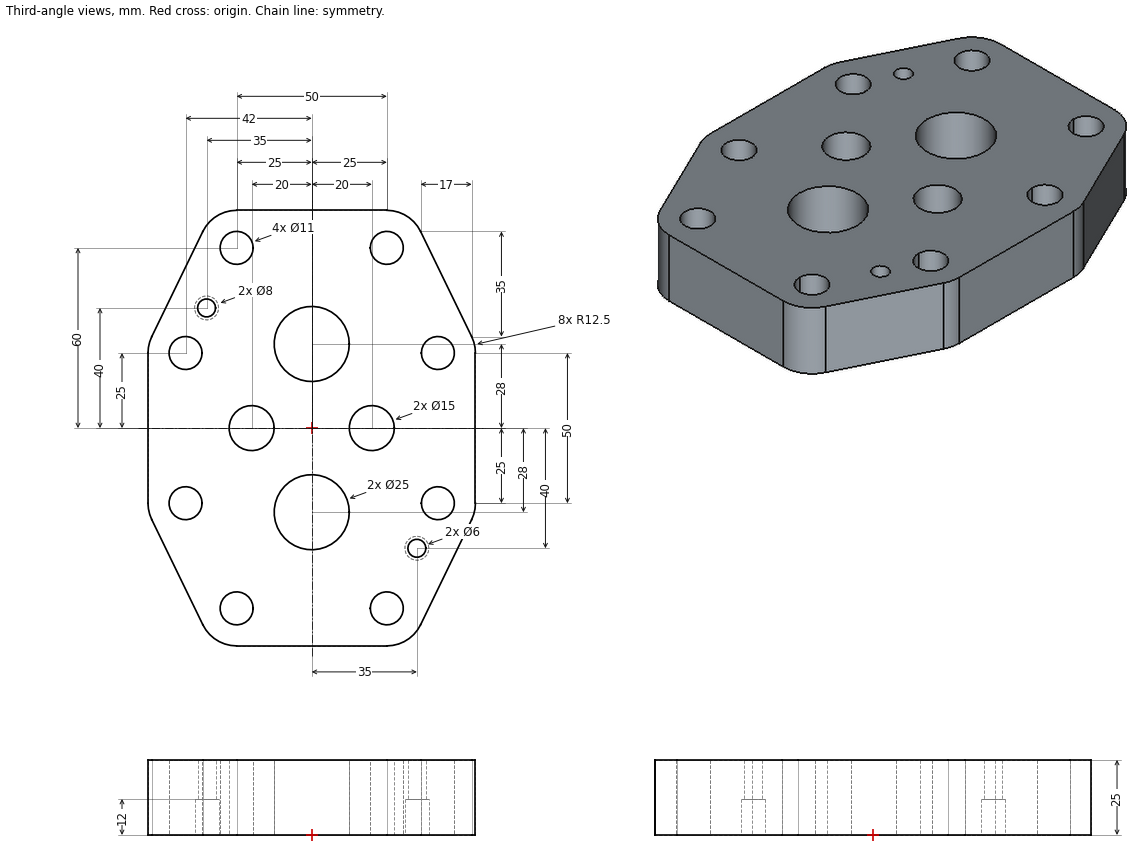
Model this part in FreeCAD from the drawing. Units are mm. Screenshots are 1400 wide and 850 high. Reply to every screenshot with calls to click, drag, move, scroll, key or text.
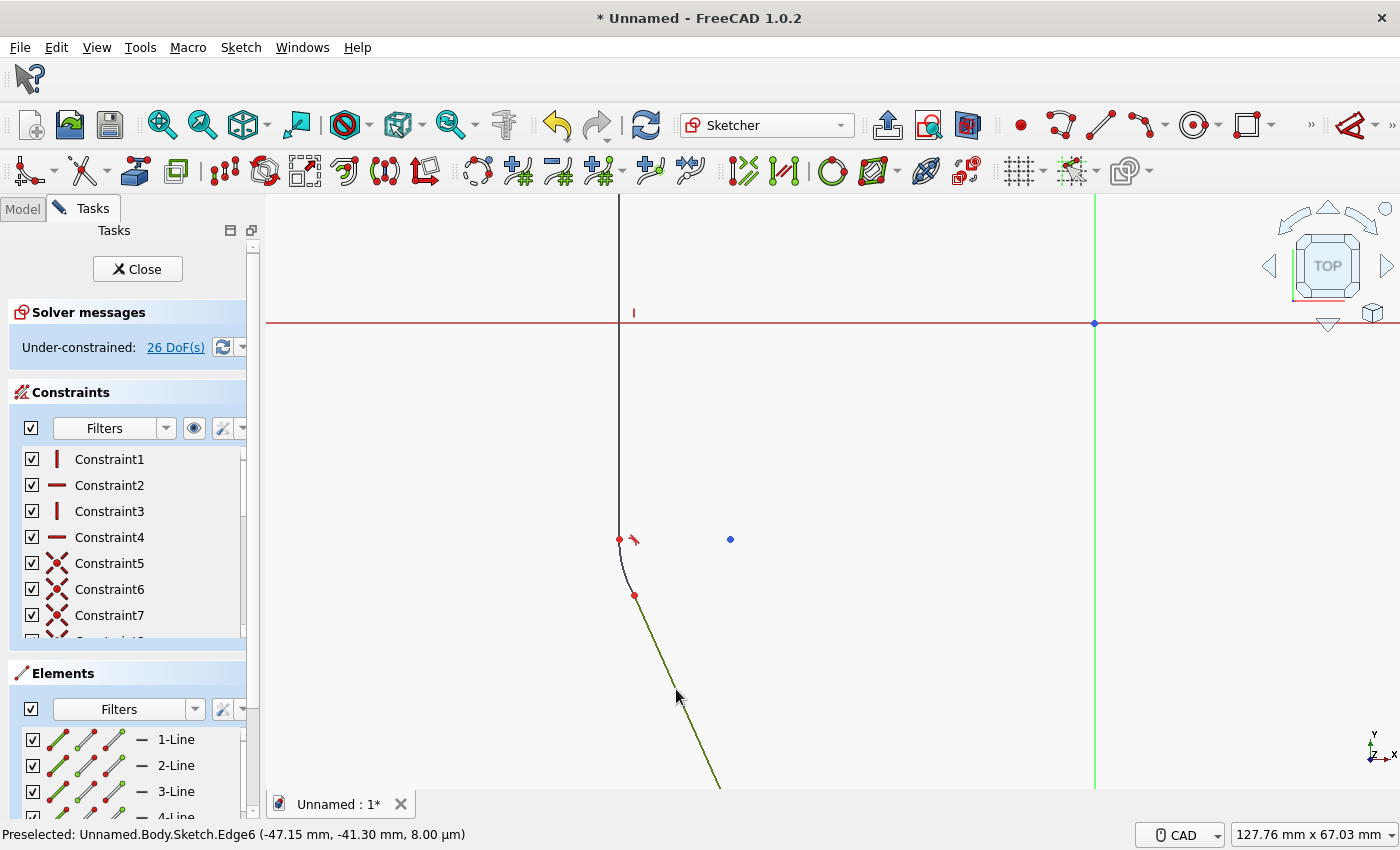
click(621, 557)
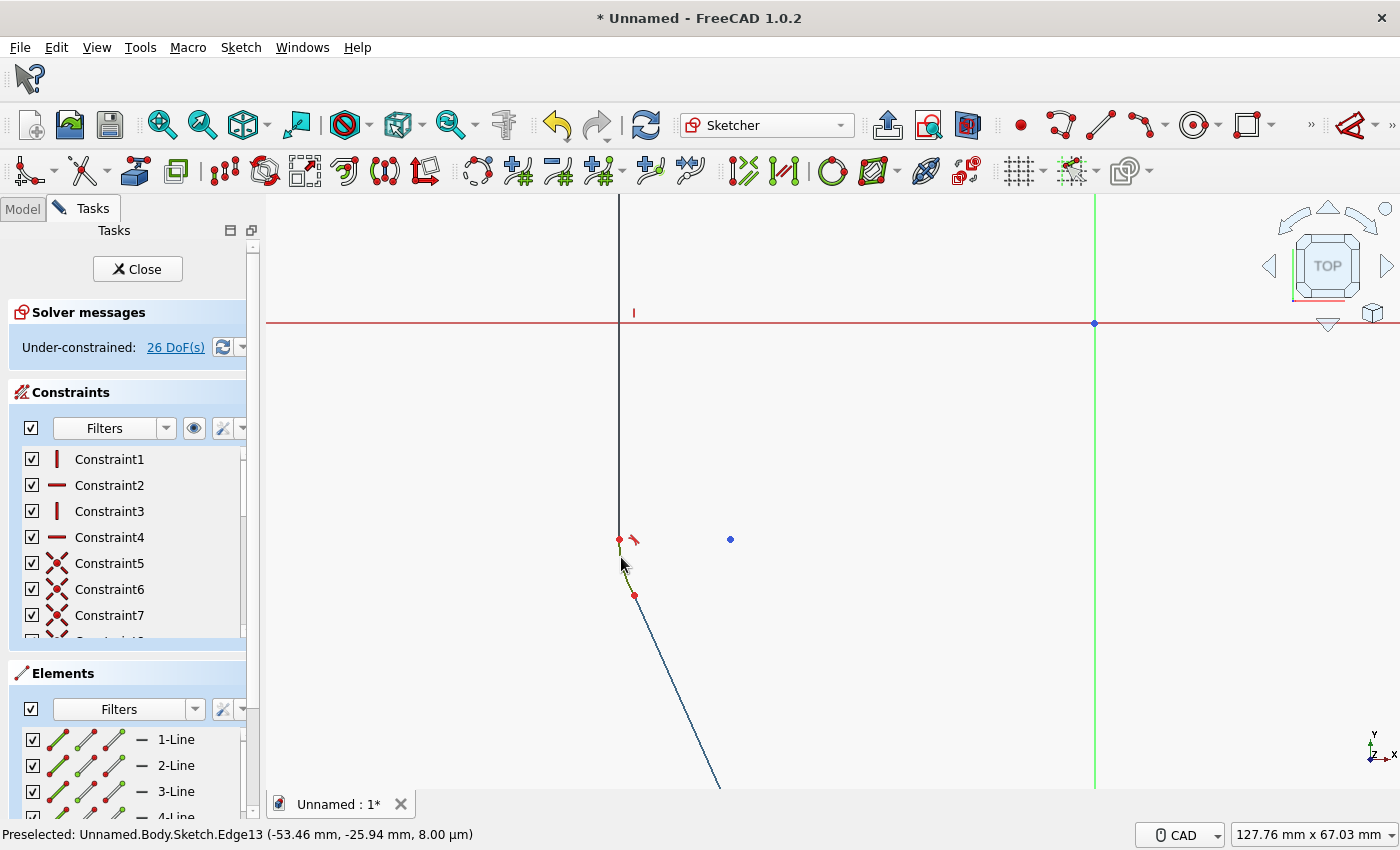
key(t)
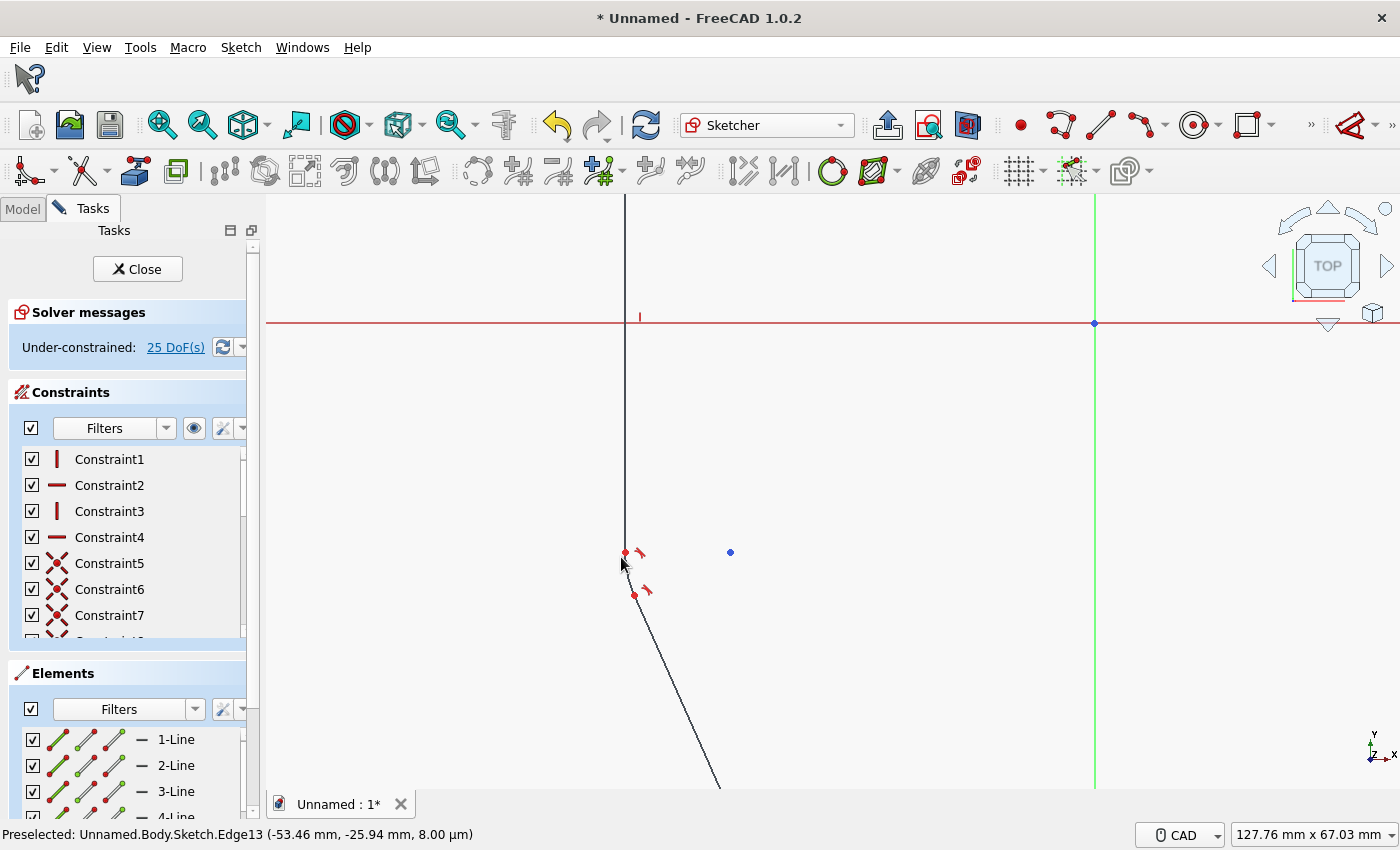
click(676, 689)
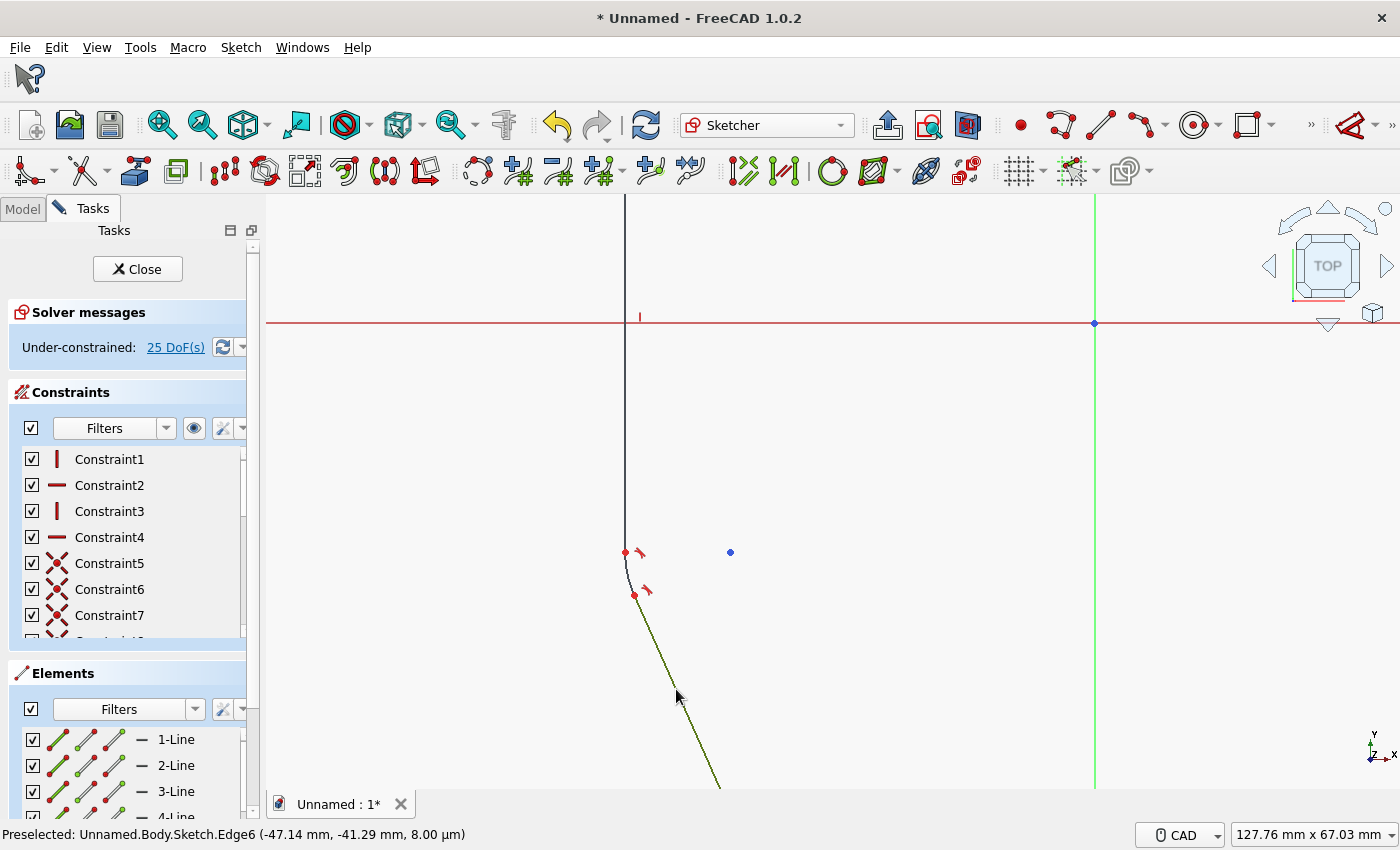
scroll(622, 564, down, 6)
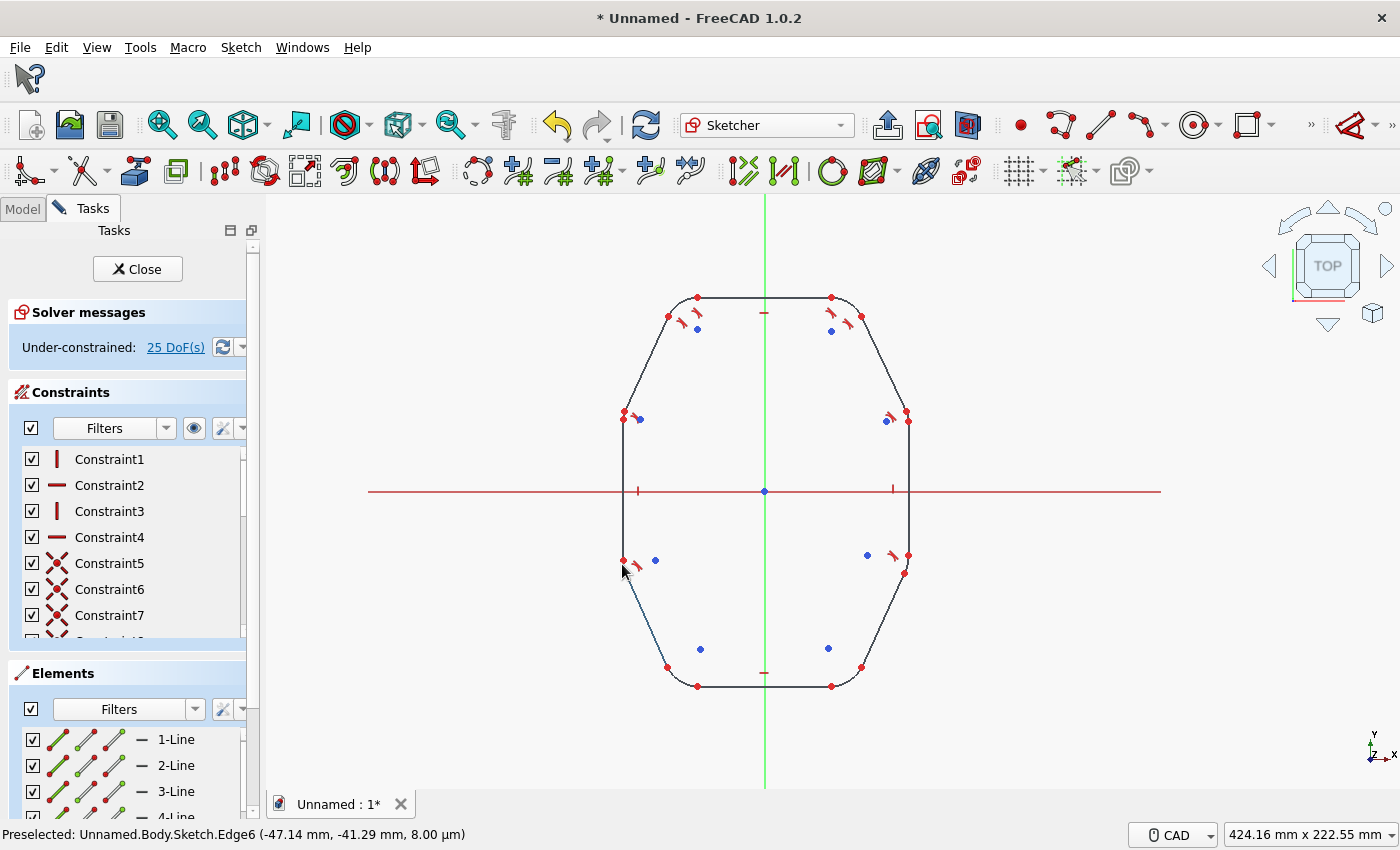
scroll(674, 677, up, 2)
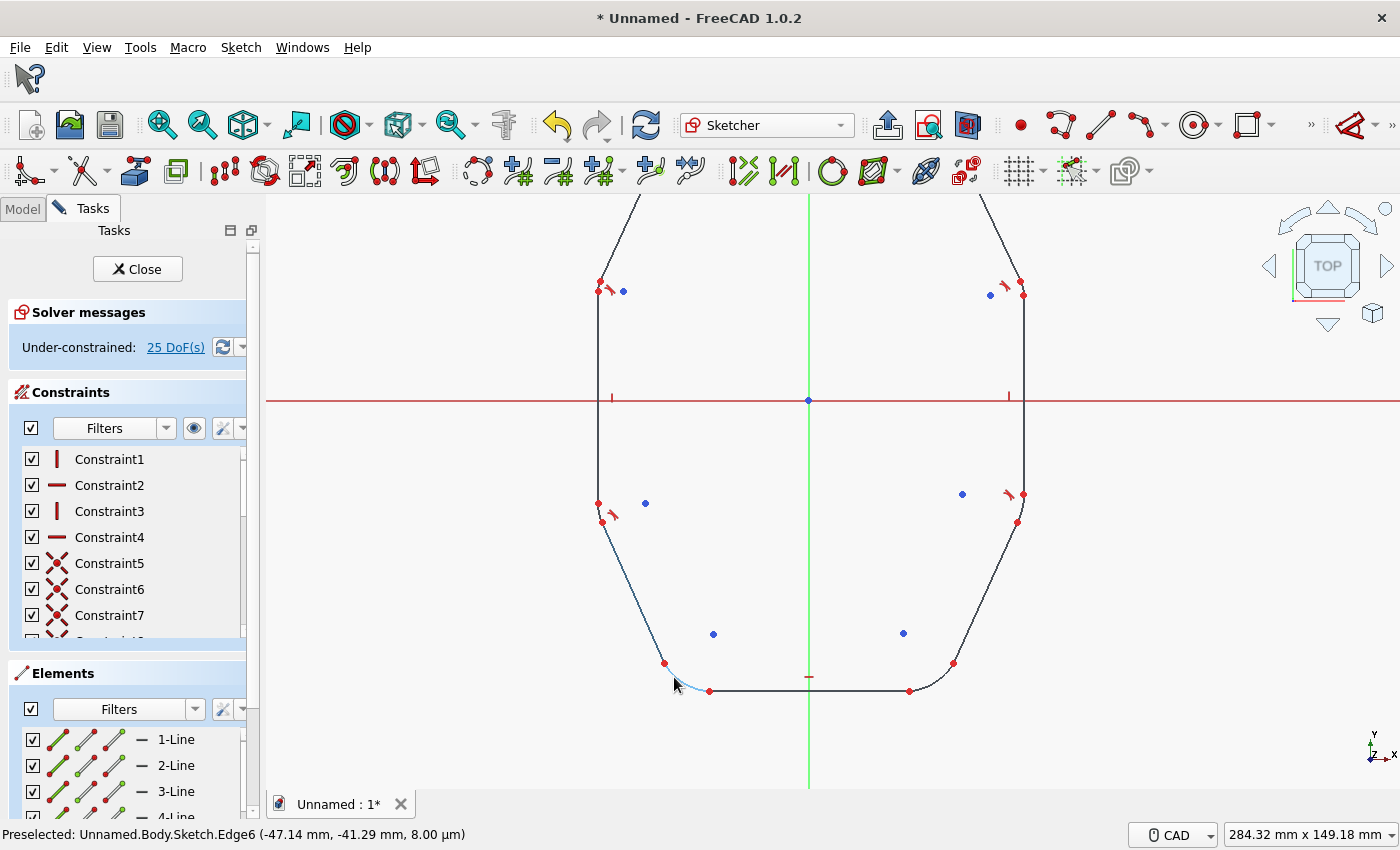
click(675, 676)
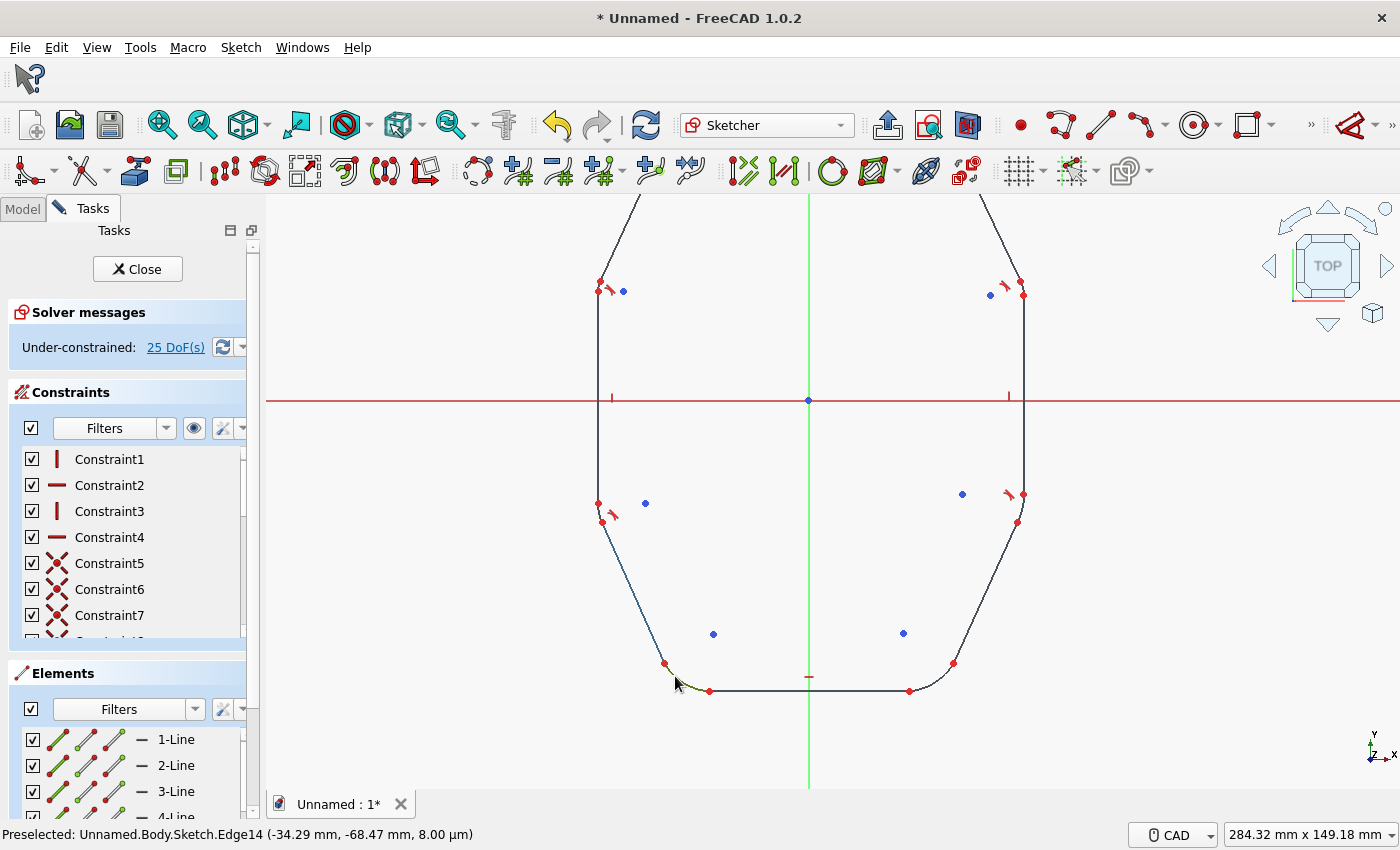
key(t)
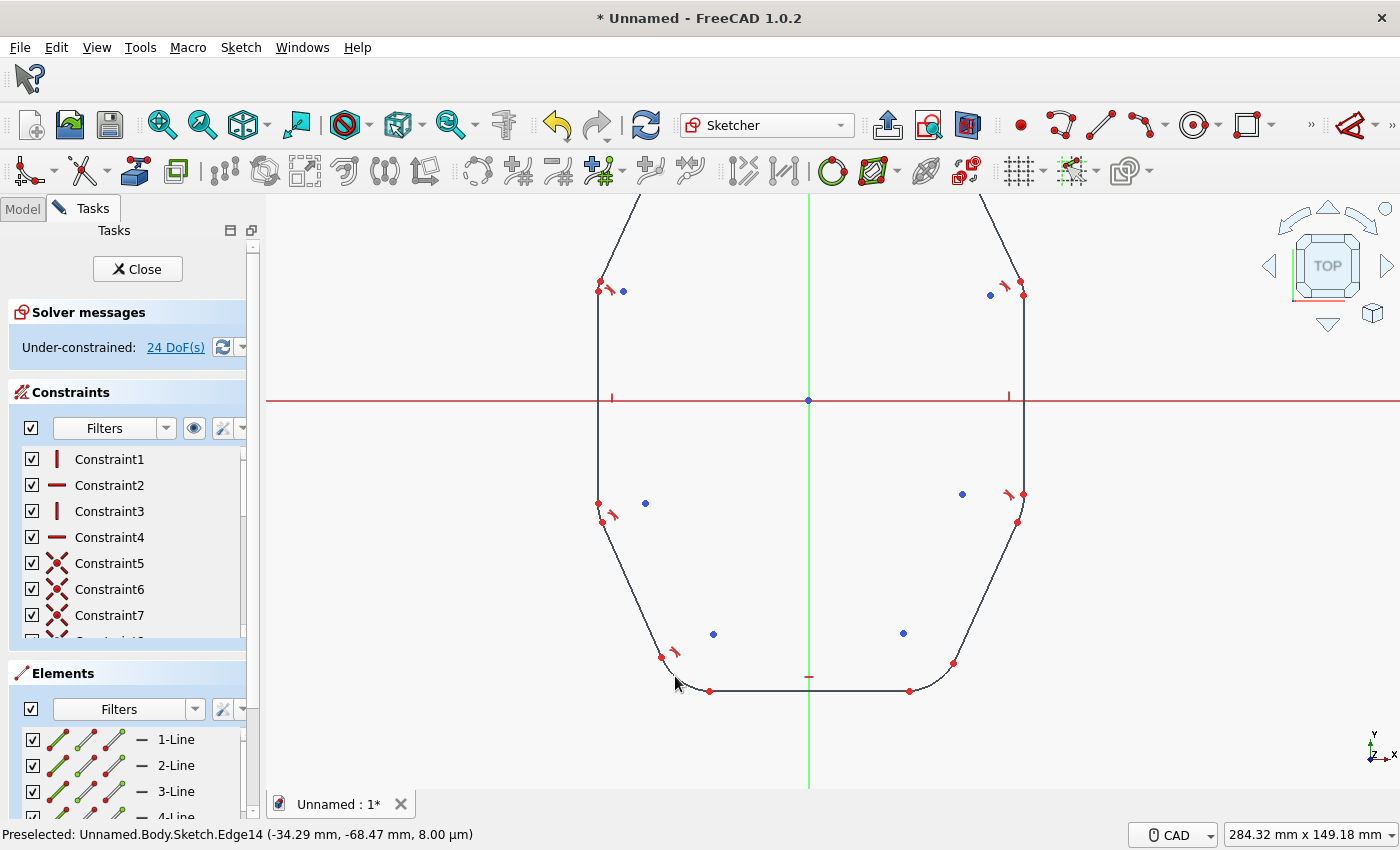
click(769, 691)